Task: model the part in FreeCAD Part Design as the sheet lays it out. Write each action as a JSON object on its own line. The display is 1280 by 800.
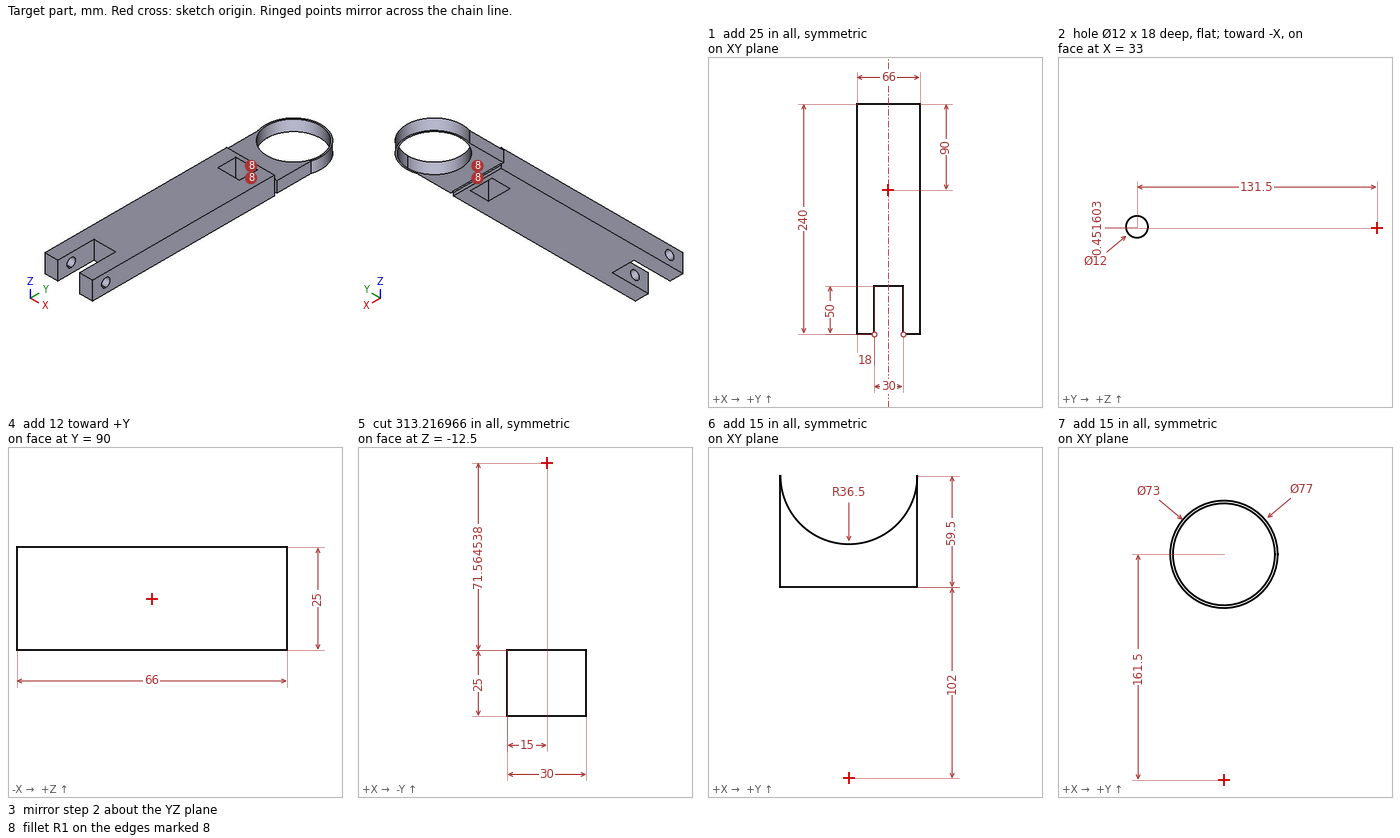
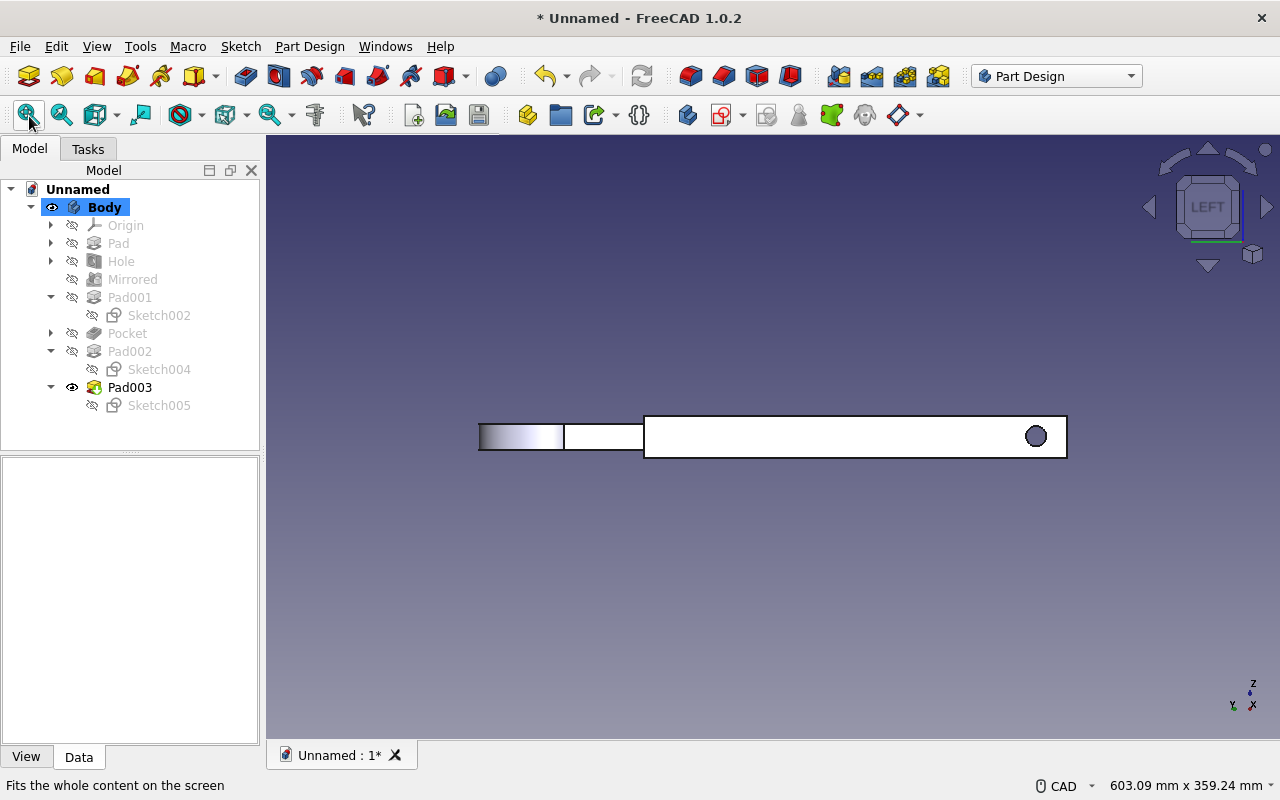
{"action": "key", "text": "v 3"}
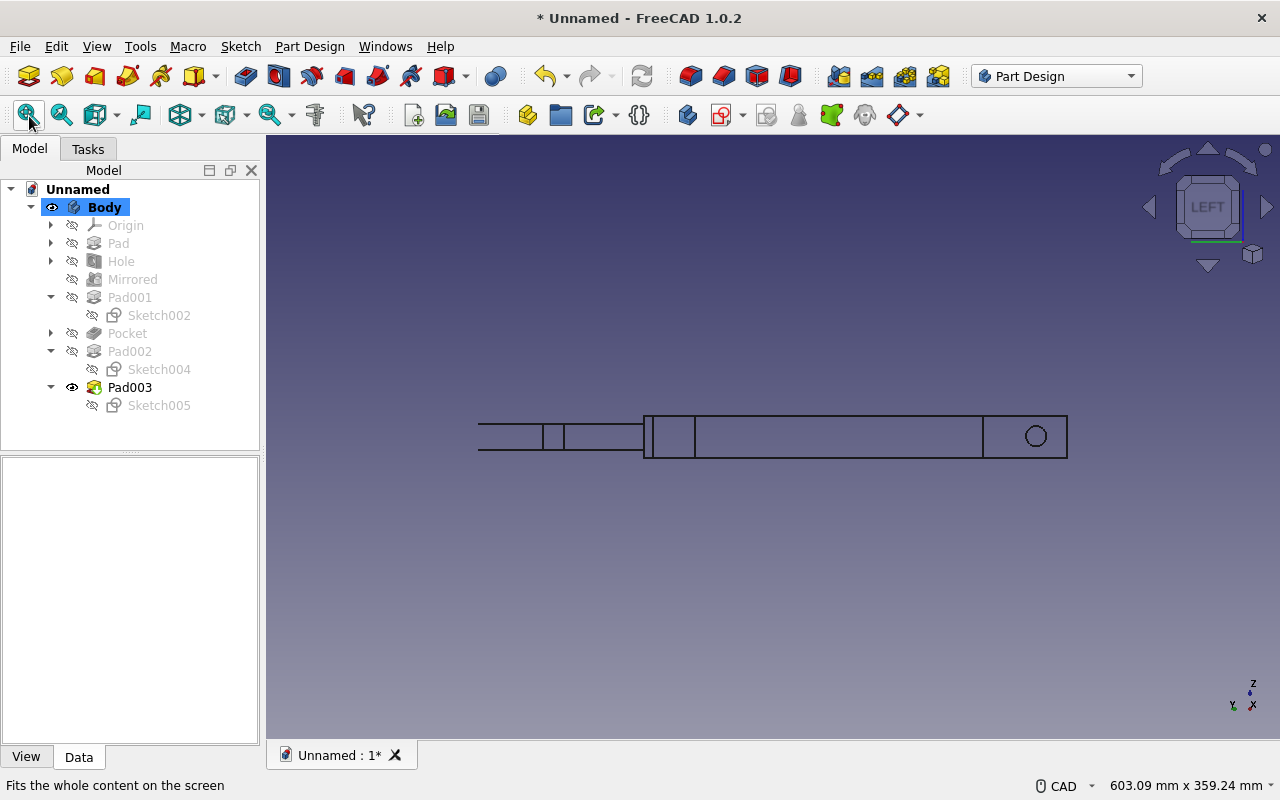
{"action": "key", "text": "0"}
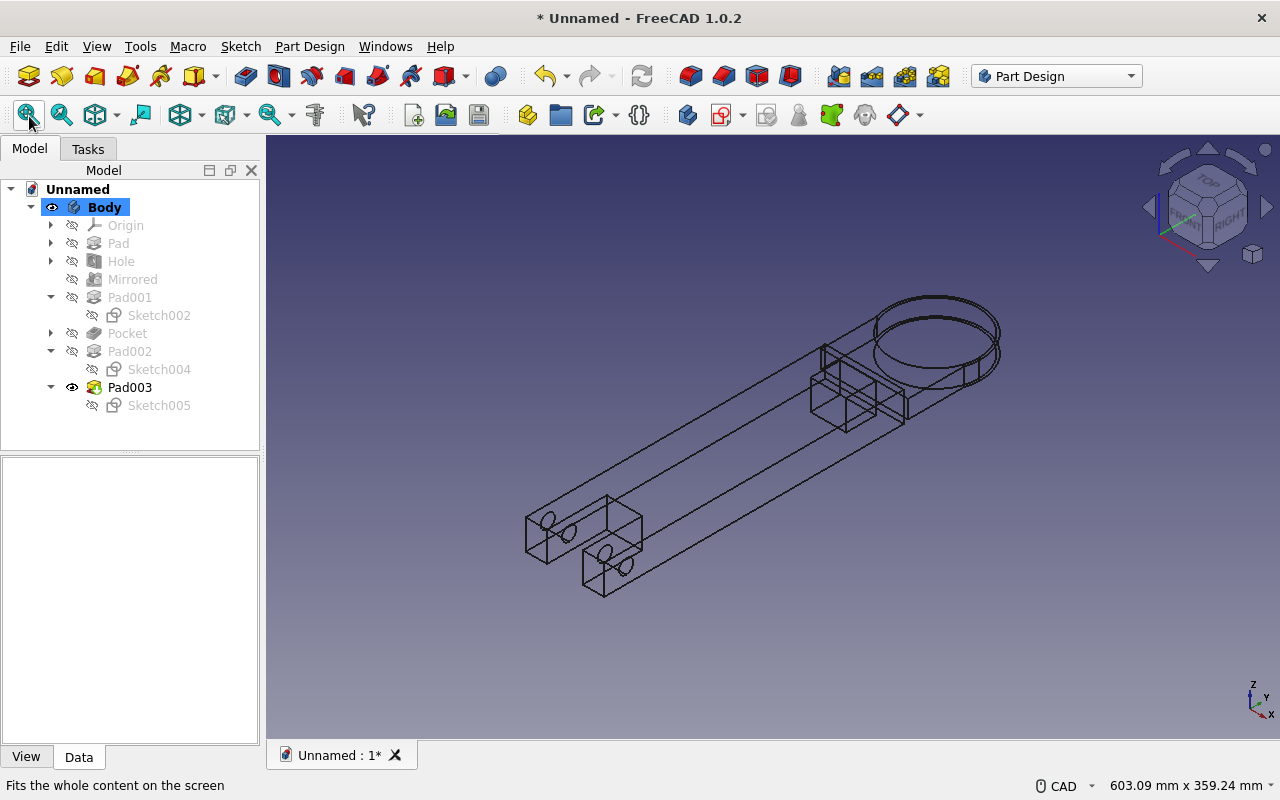
{"action": "left_click", "coordinate": [849, 384]}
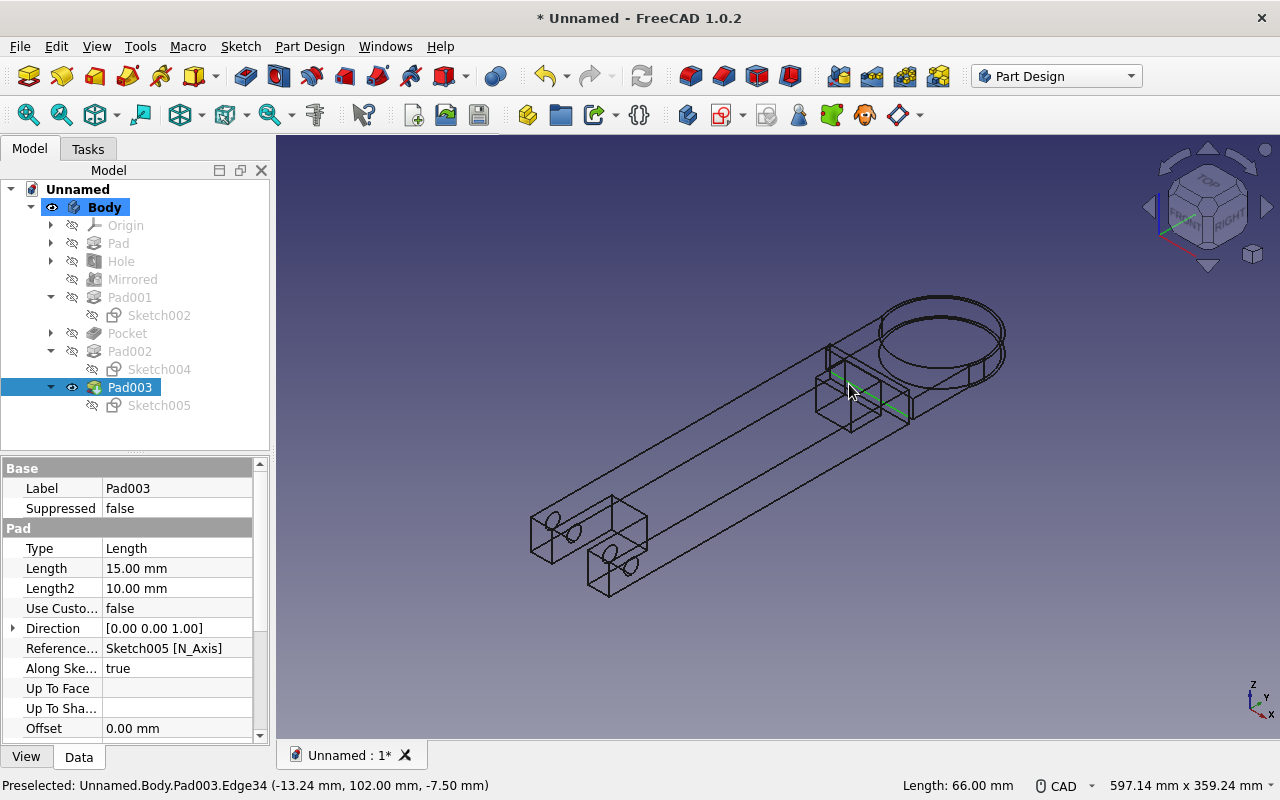
{"action": "key", "text": "2"}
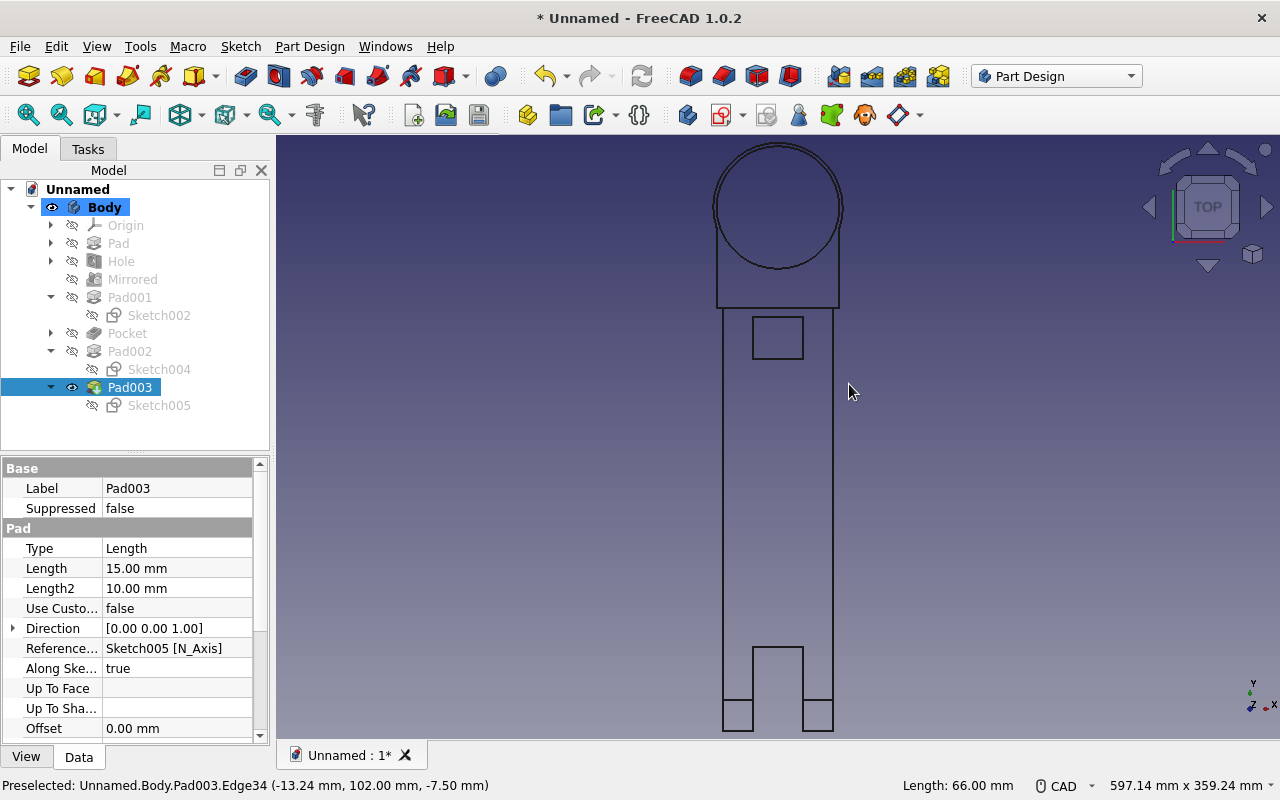
{"action": "key", "text": "1"}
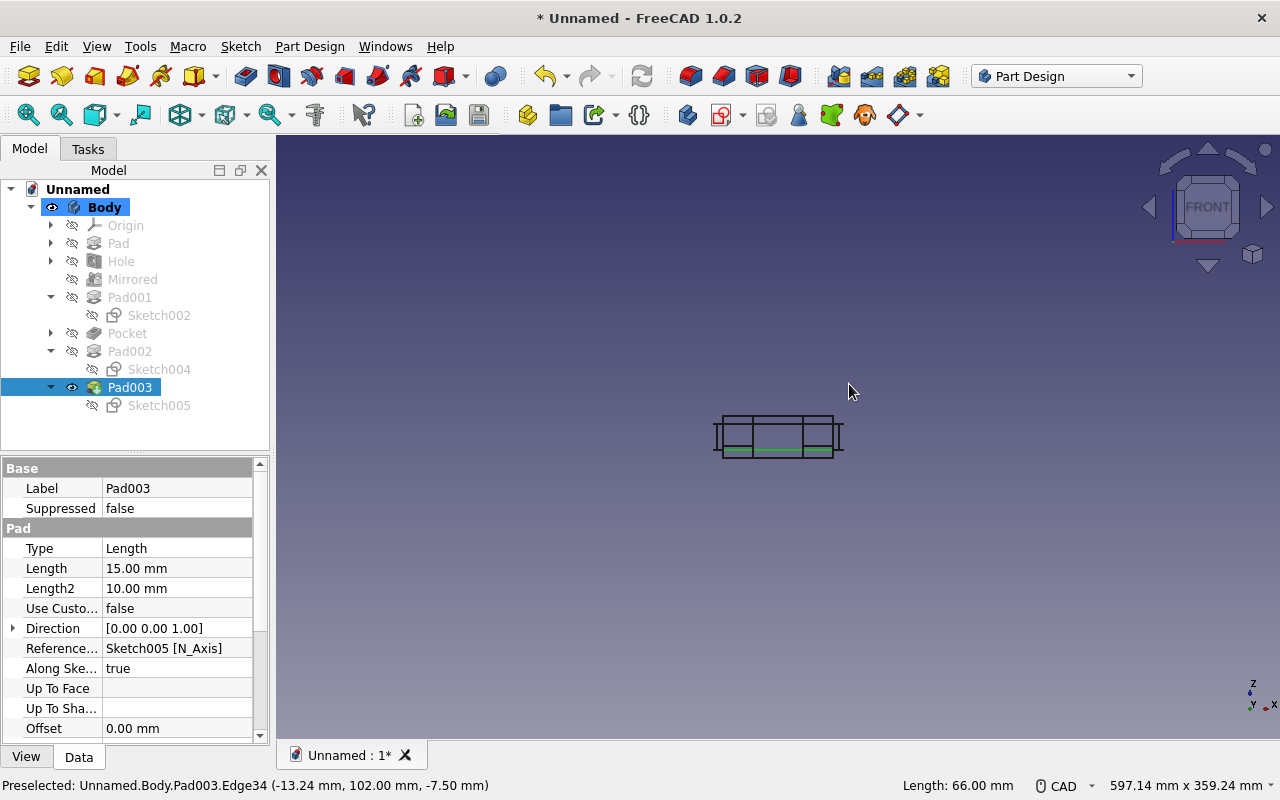
{"action": "key", "text": "v f"}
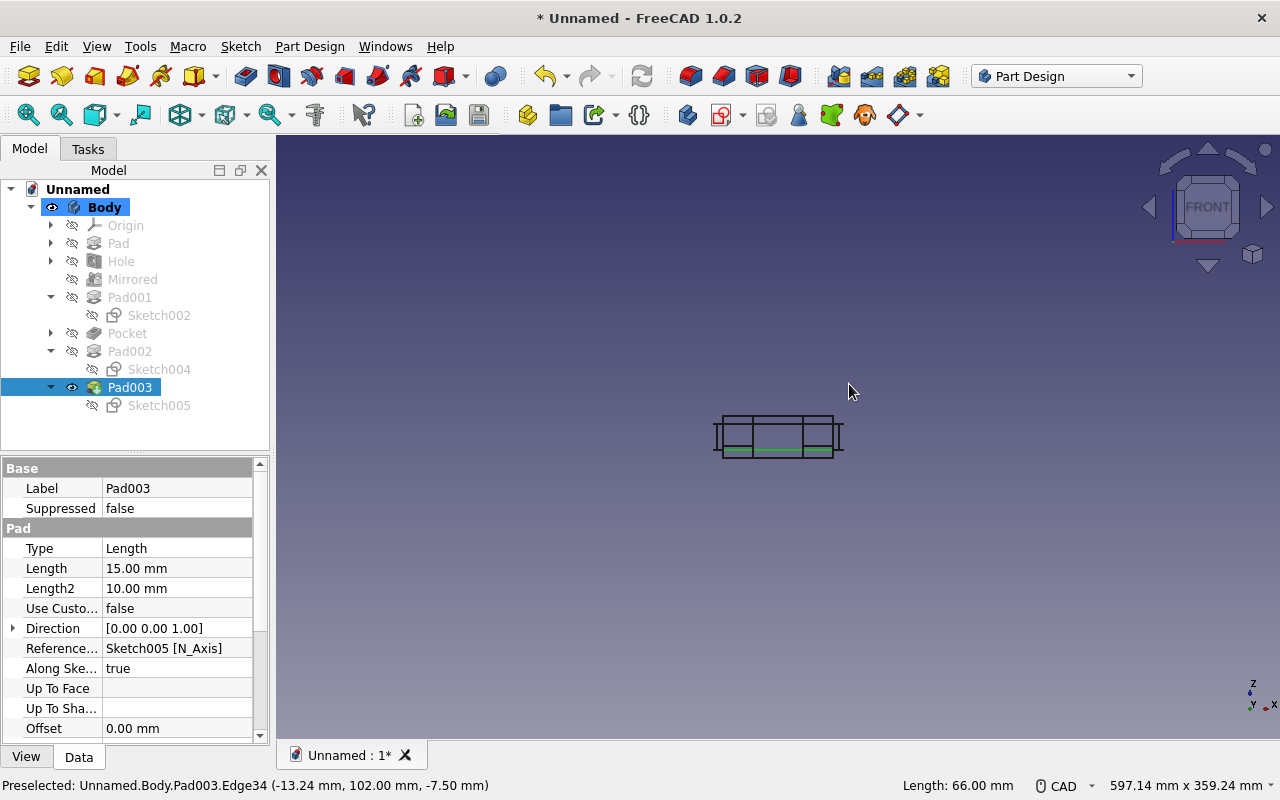
{"action": "left_click", "coordinate": [778, 423], "text": "ctrl"}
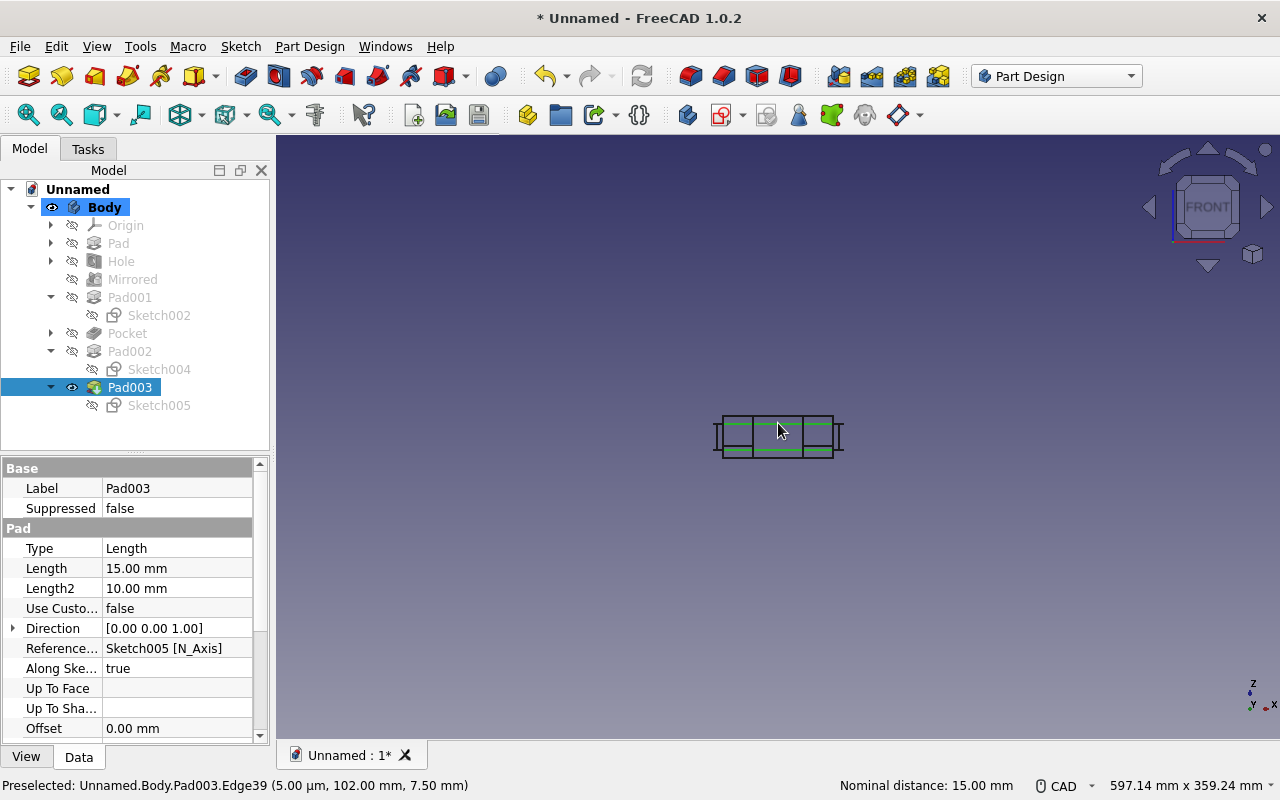
{"action": "key", "text": "v 1"}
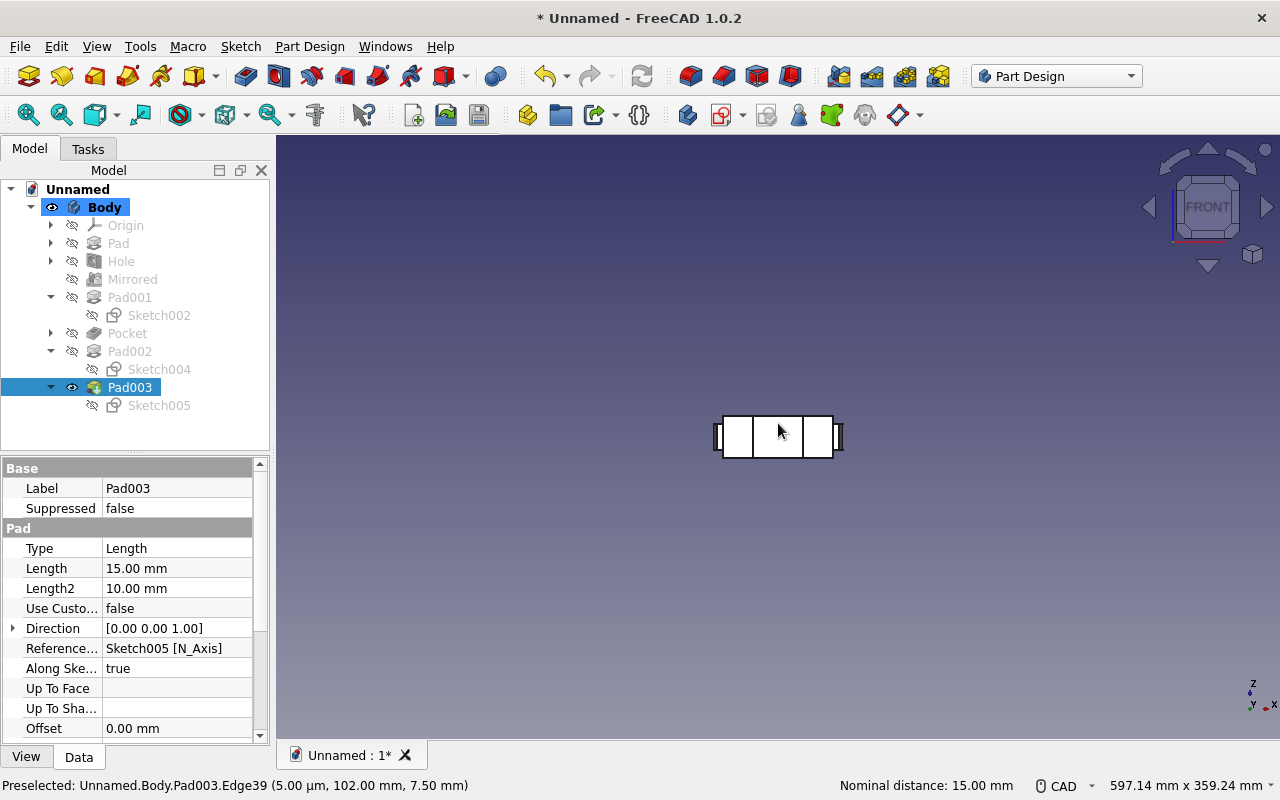
{"action": "left_click", "coordinate": [691, 76]}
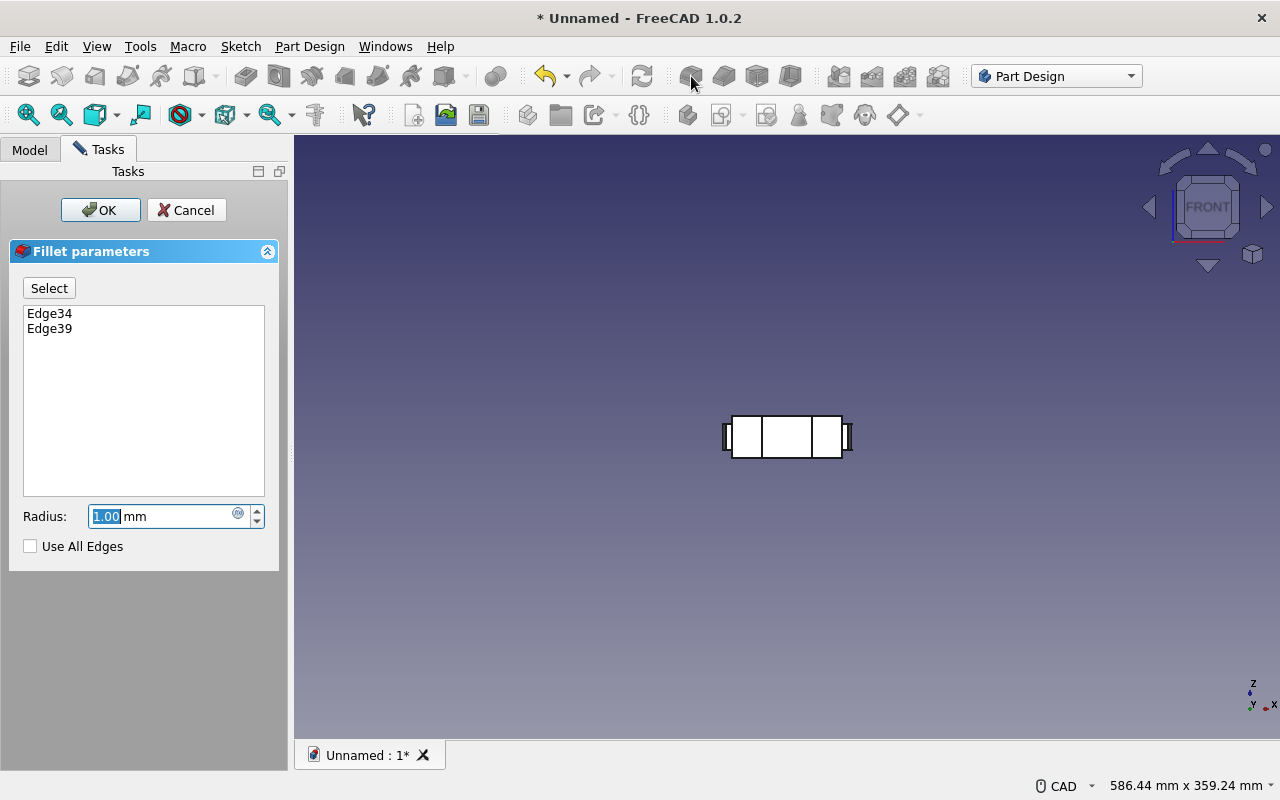
{"action": "type", "text": "1"}
{"action": "key", "text": "Tab"}